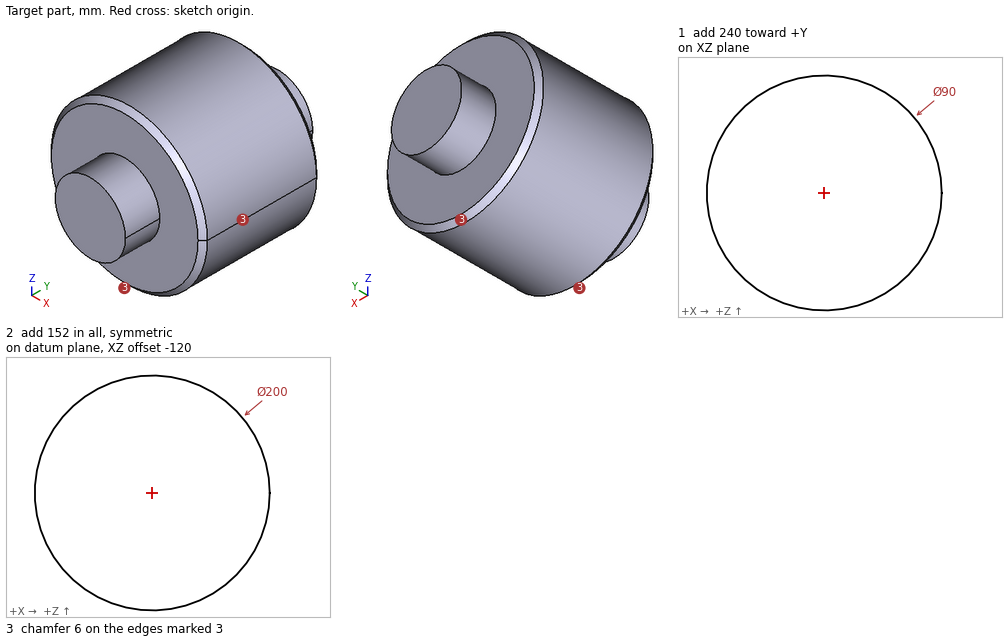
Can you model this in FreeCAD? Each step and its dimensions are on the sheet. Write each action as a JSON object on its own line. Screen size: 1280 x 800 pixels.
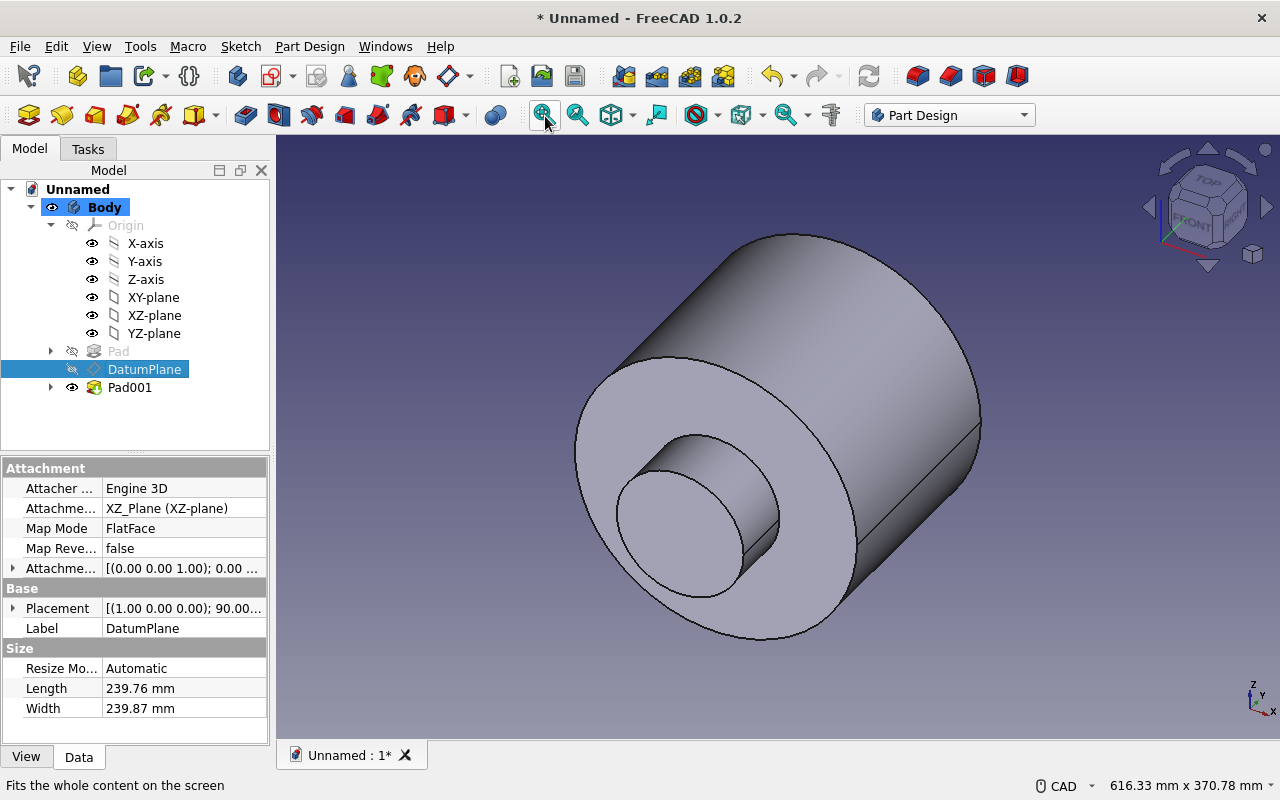
{"action": "left_click", "coordinate": [602, 381]}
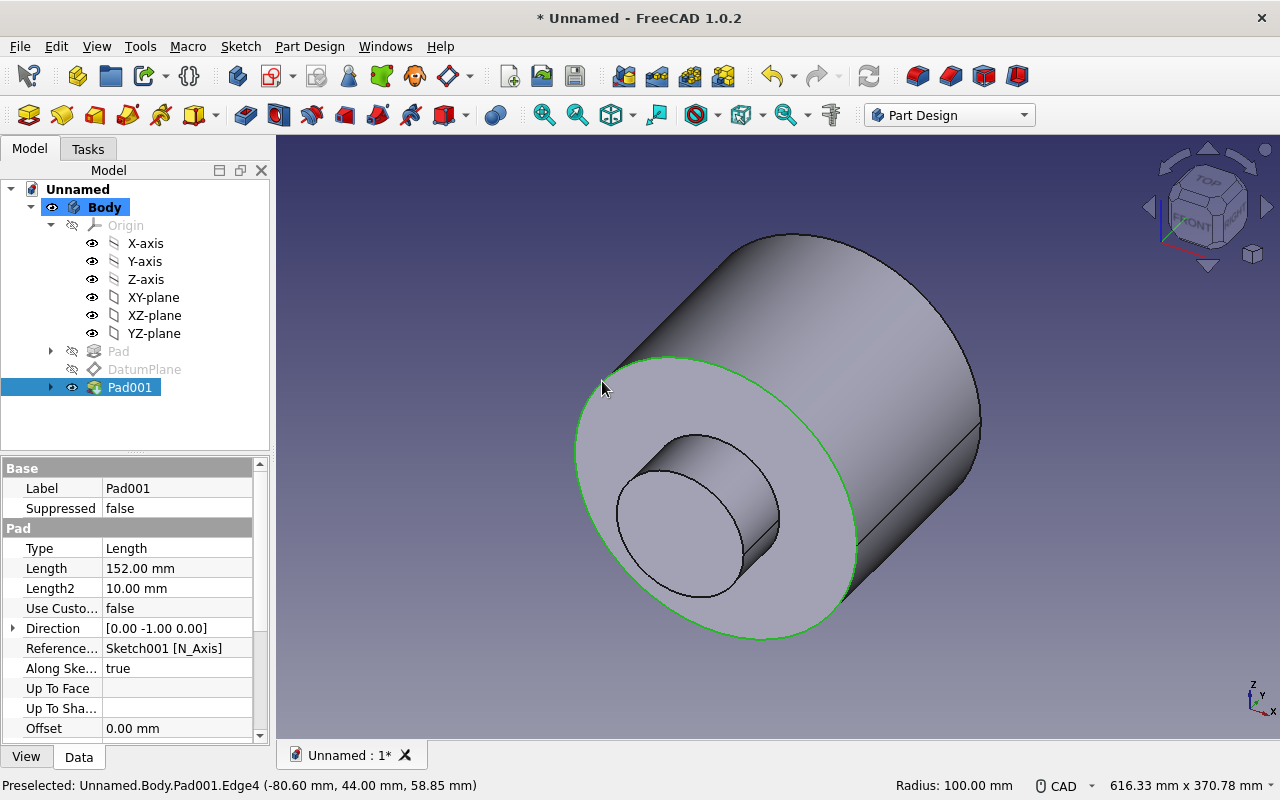
{"action": "key", "text": "0"}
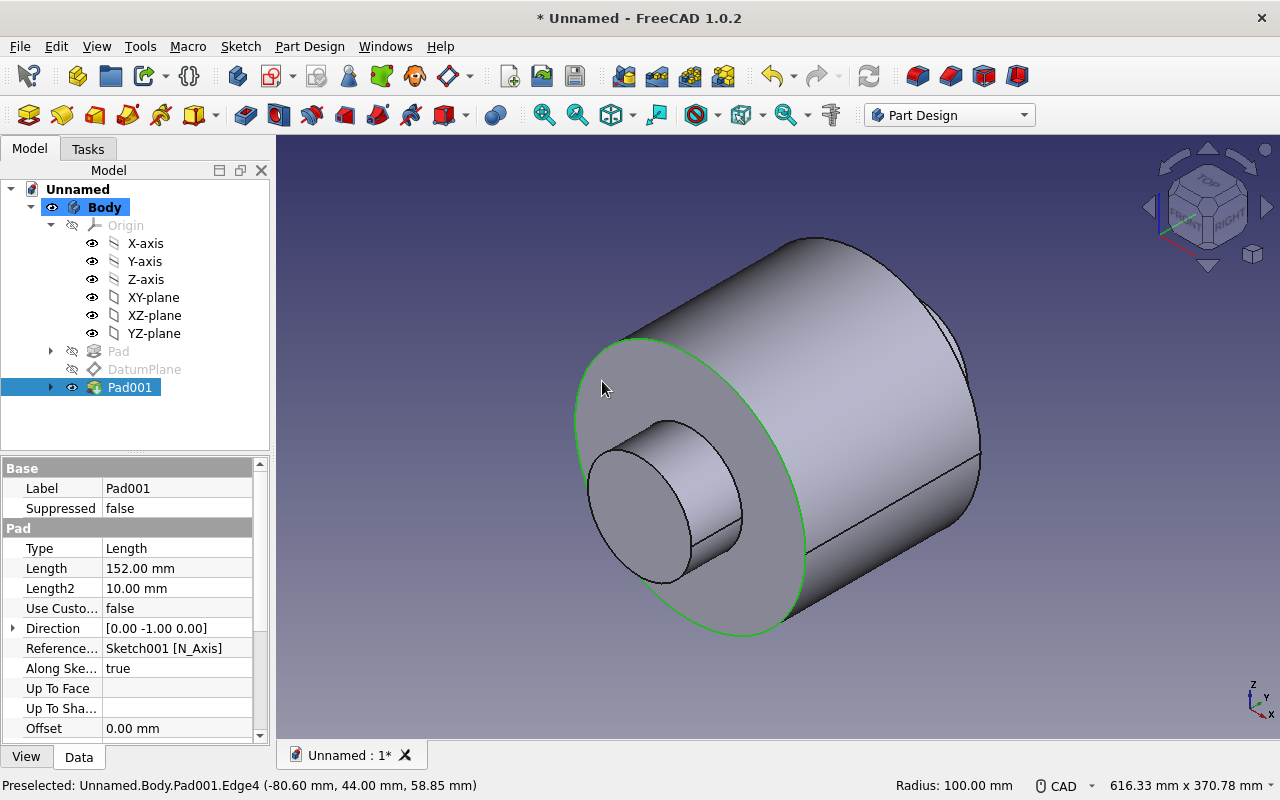
{"action": "key", "text": "2"}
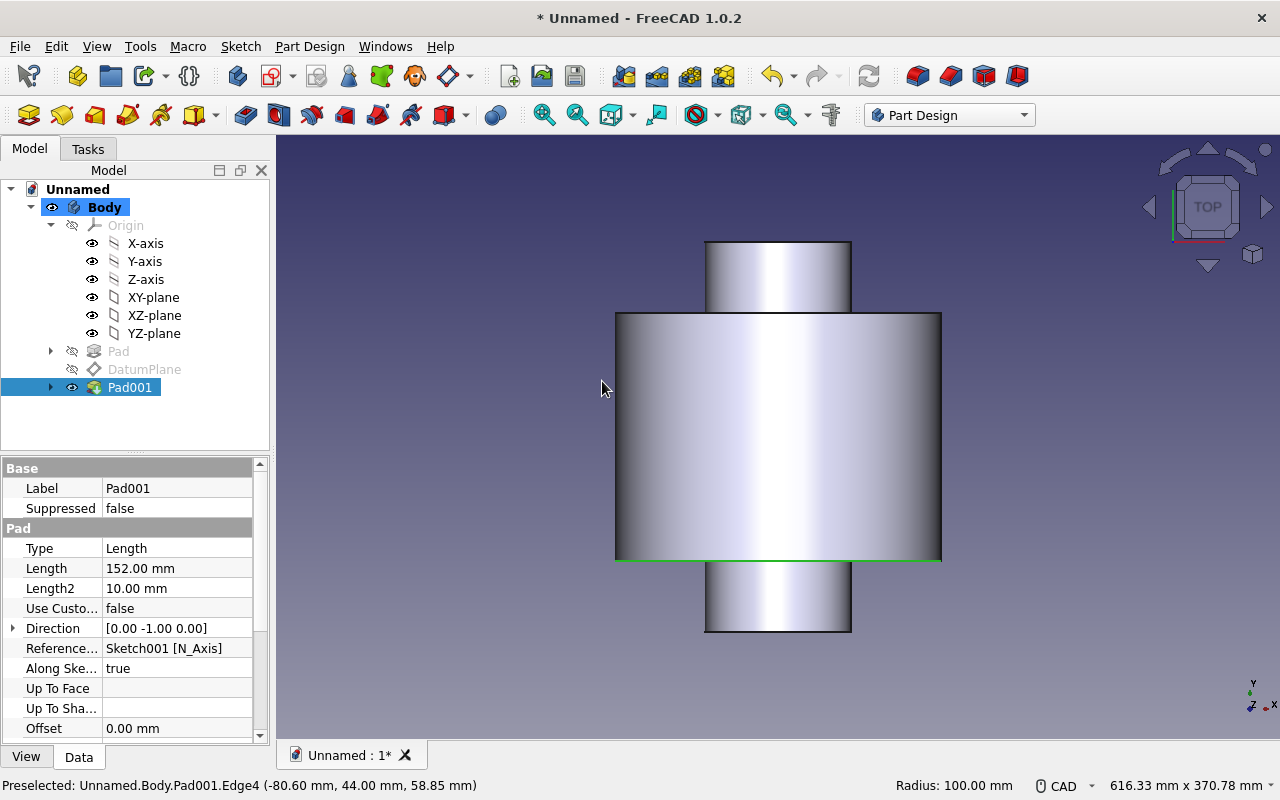
{"action": "left_click", "coordinate": [646, 312], "text": "ctrl"}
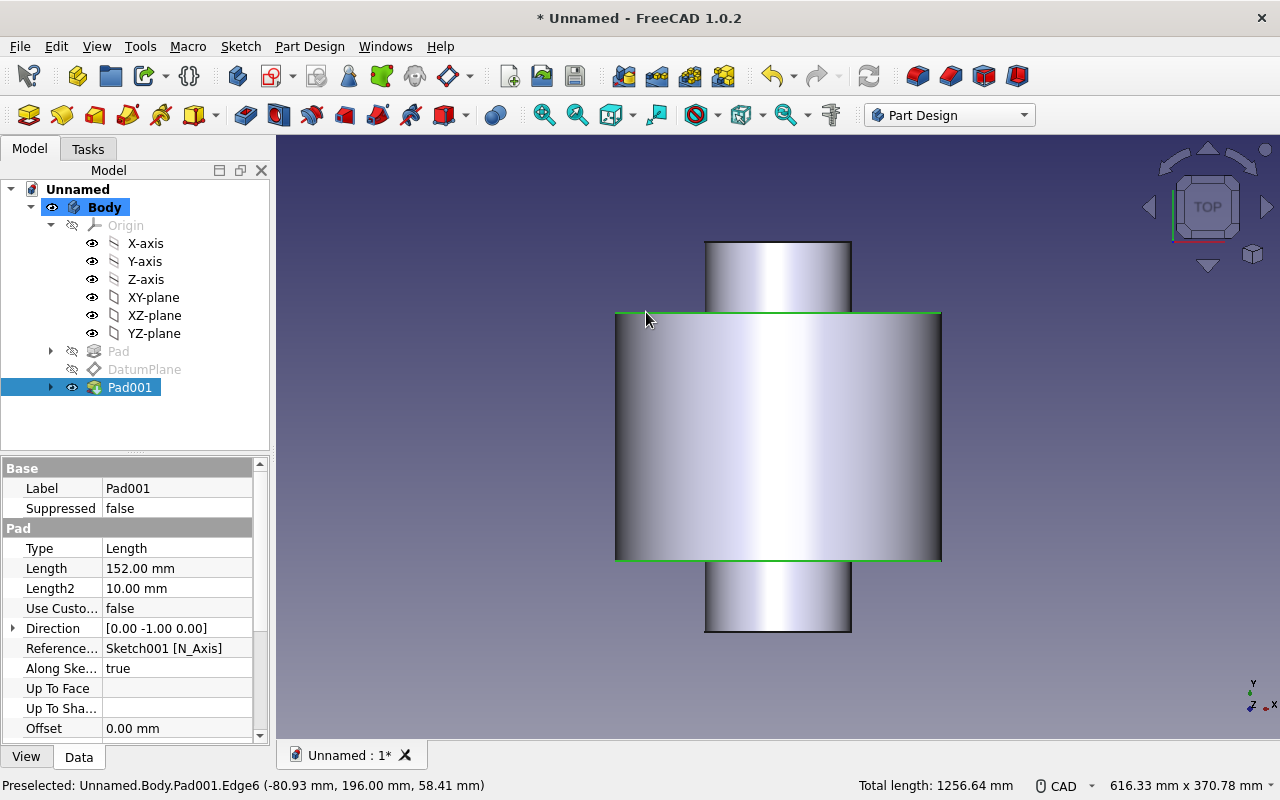
{"action": "left_click", "coordinate": [951, 76]}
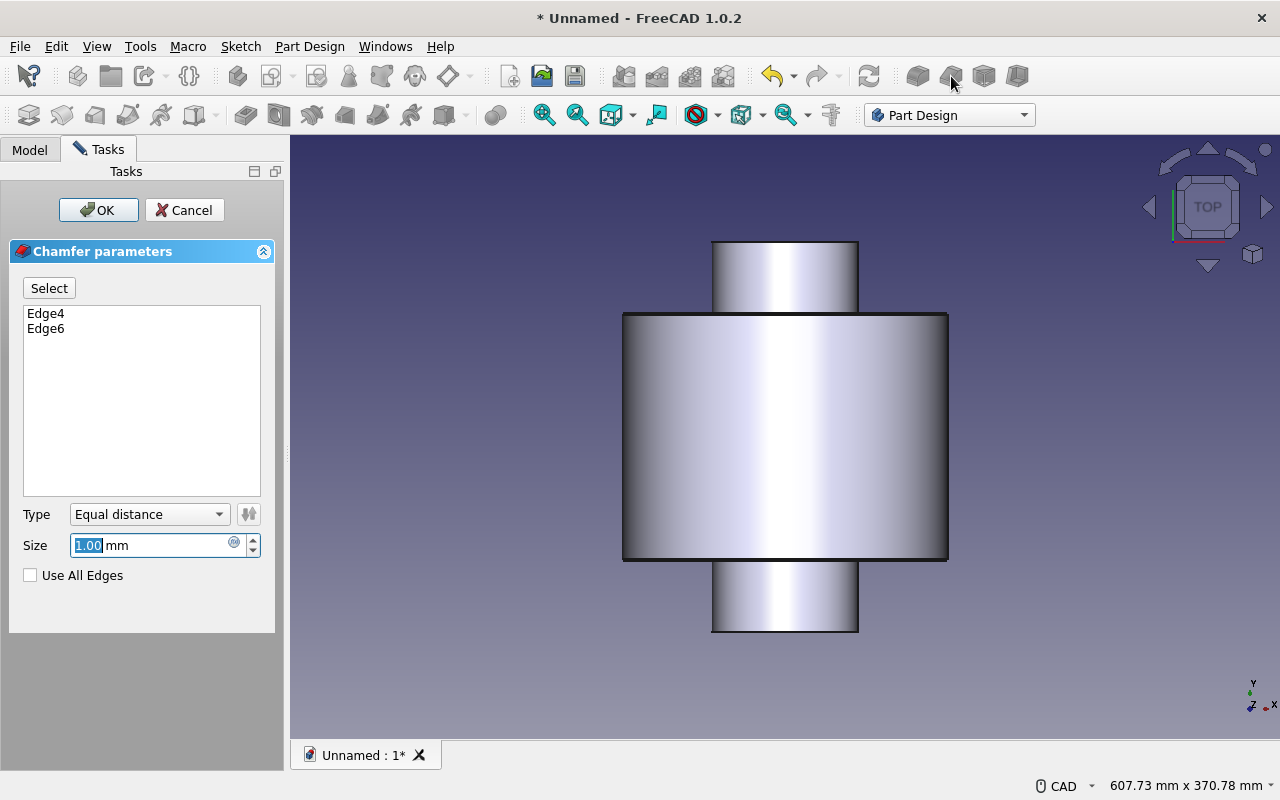
{"action": "type", "text": "6"}
{"action": "key", "text": "Tab"}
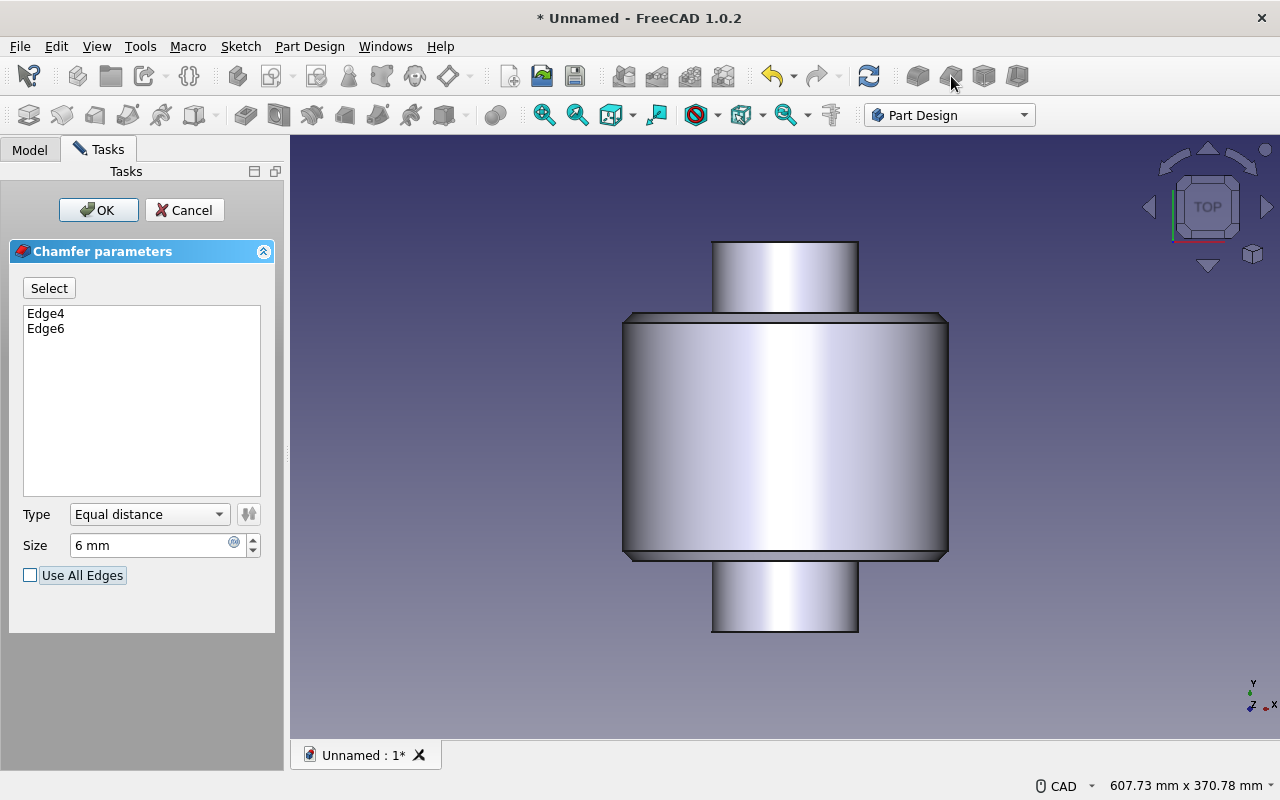
{"action": "left_click", "coordinate": [99, 210]}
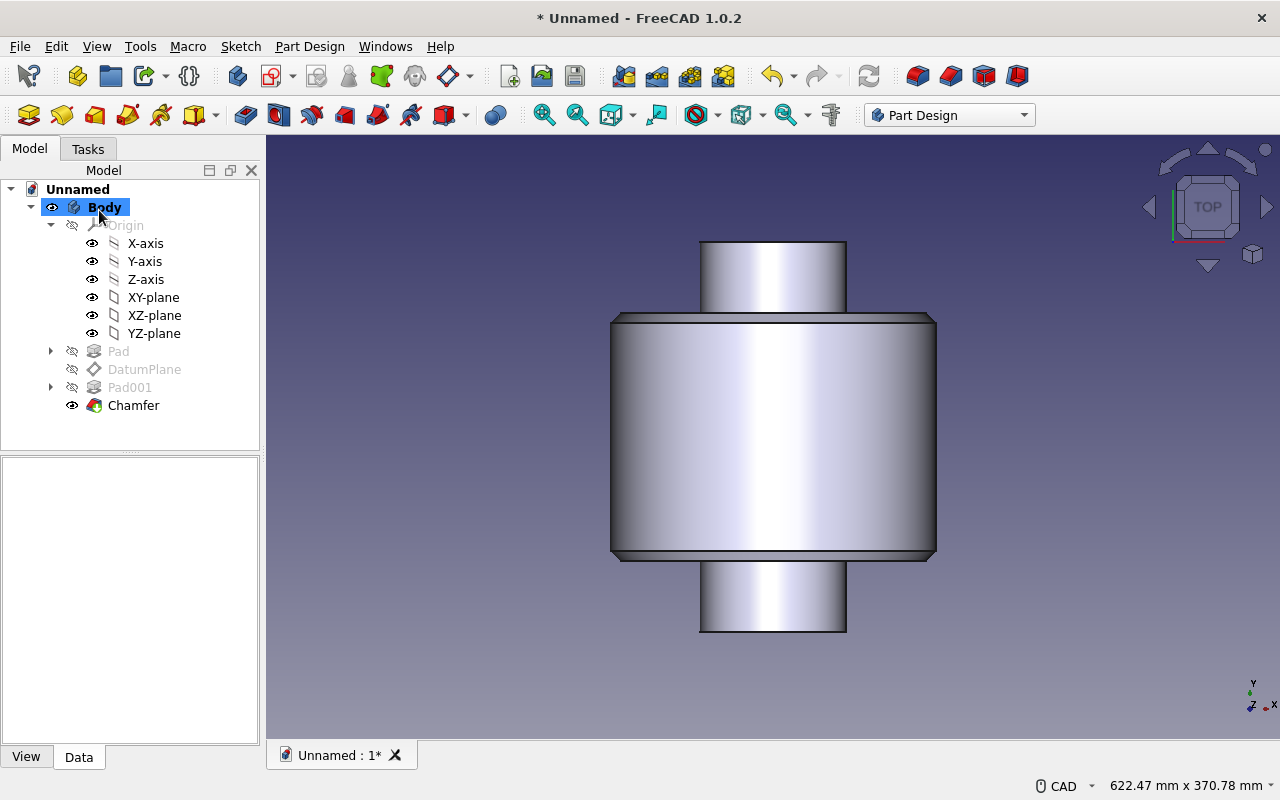
{"action": "key", "text": "0"}